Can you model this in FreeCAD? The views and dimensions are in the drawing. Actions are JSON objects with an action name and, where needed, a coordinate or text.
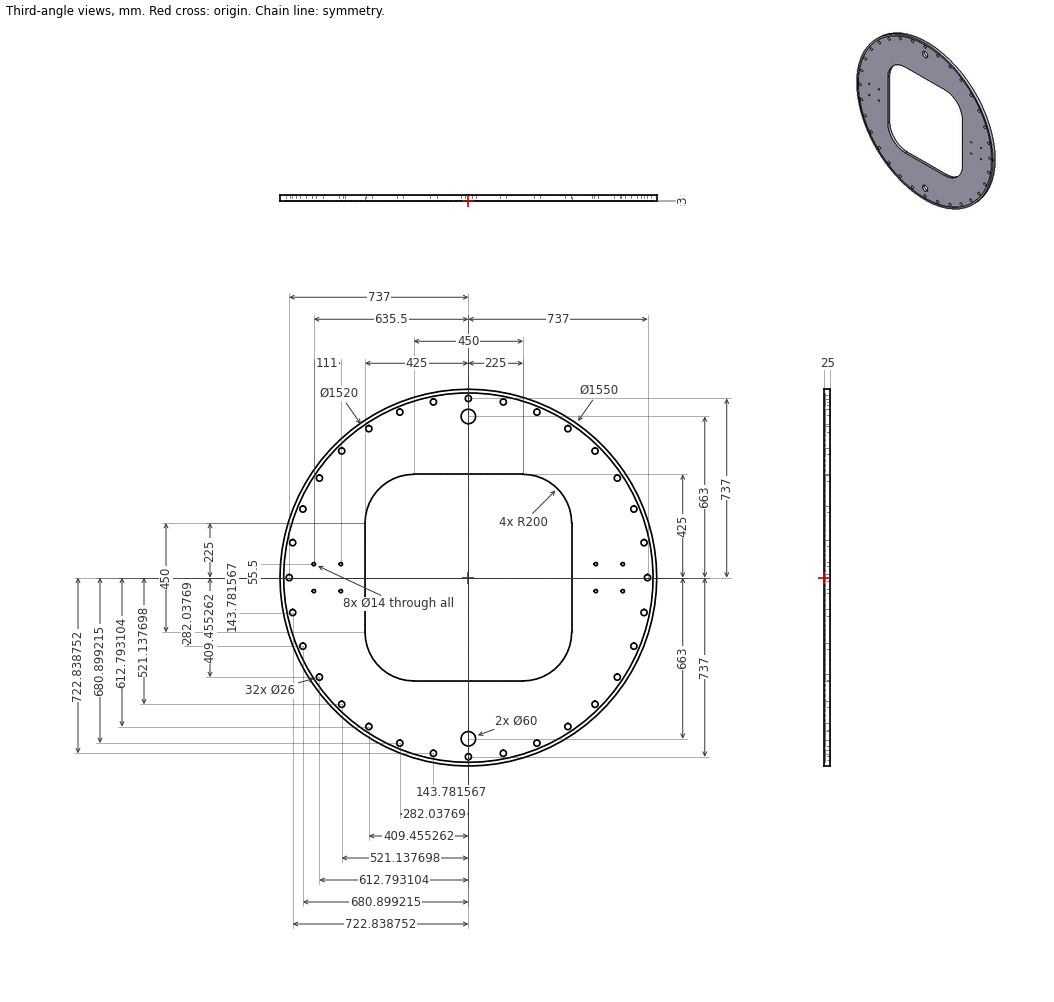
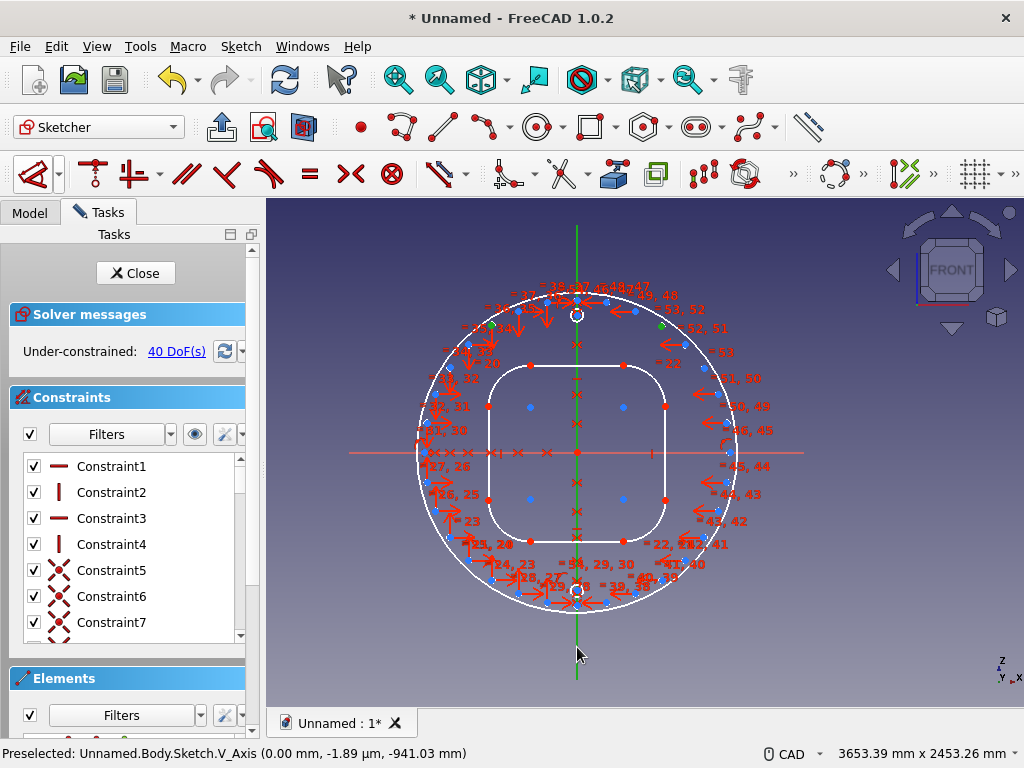
{"action": "left_click", "coordinate": [351, 174]}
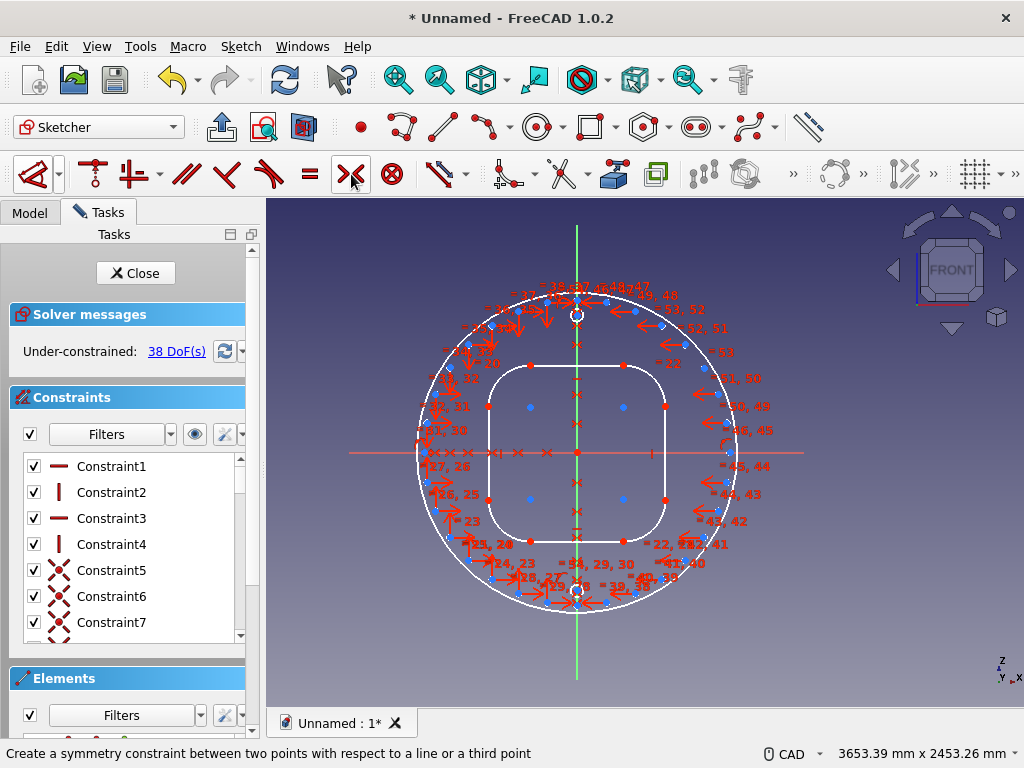
{"action": "left_click", "coordinate": [450, 368]}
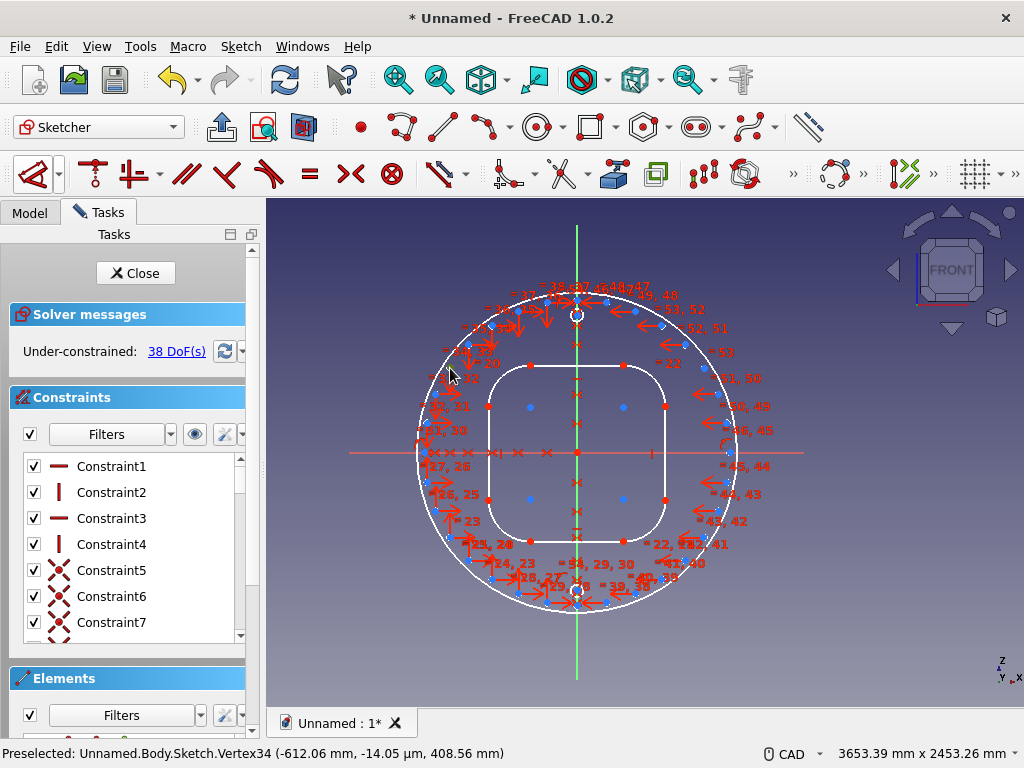
{"action": "left_click", "coordinate": [704, 368]}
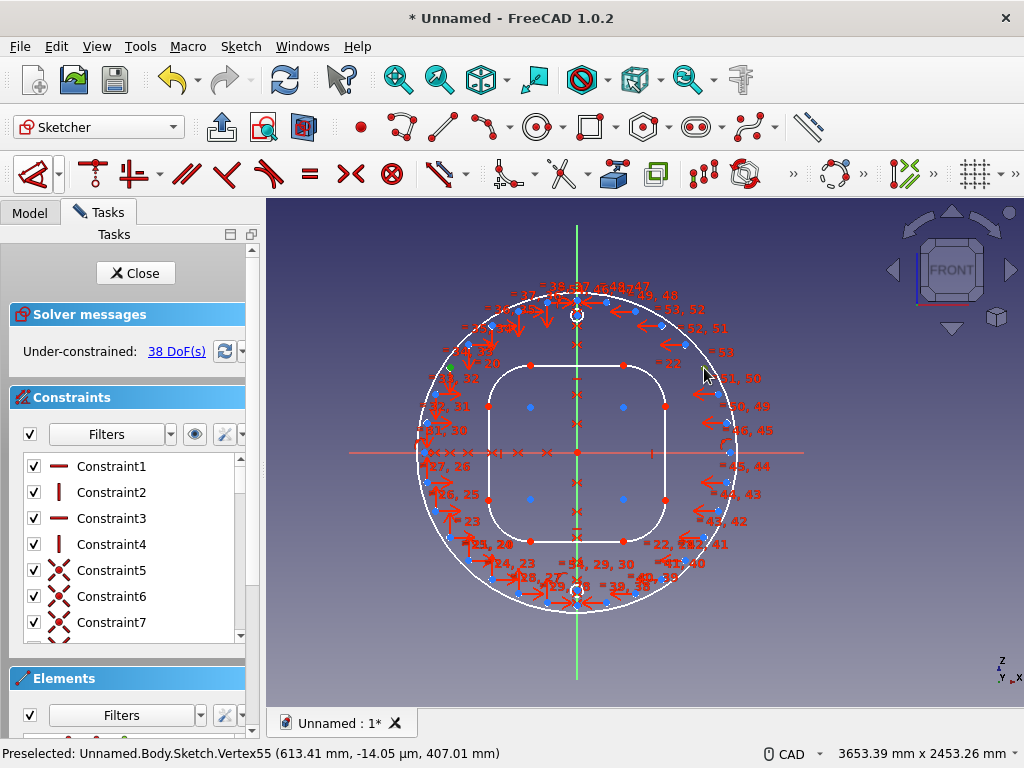
{"action": "left_click", "coordinate": [577, 647]}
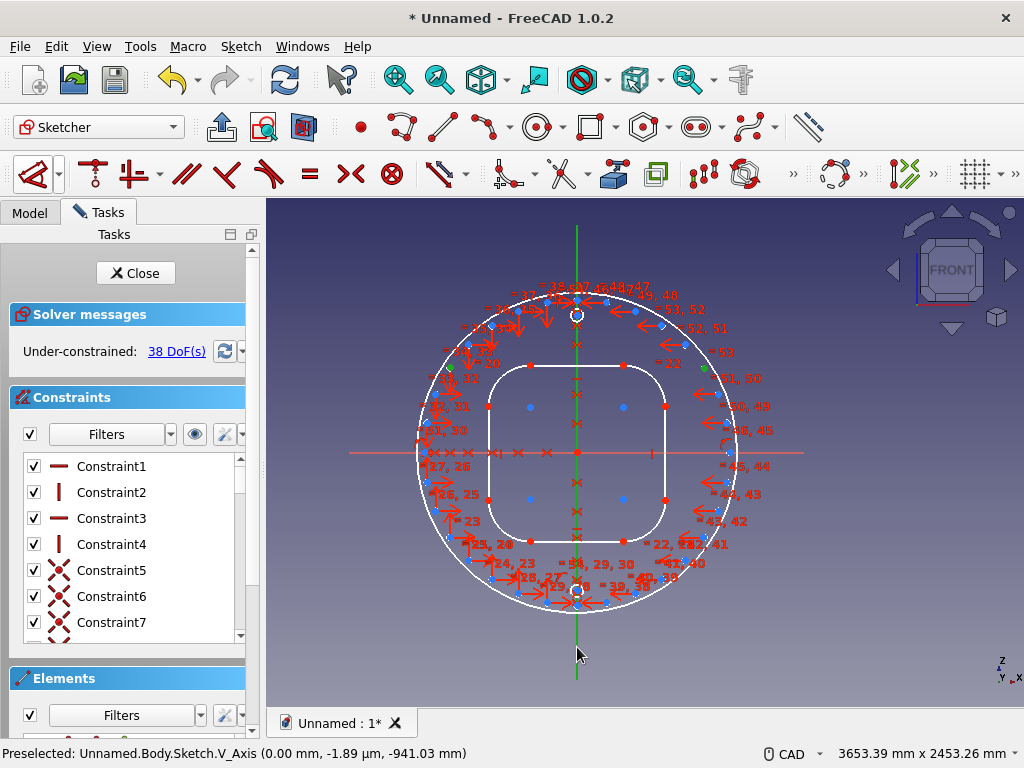
{"action": "left_click", "coordinate": [351, 174]}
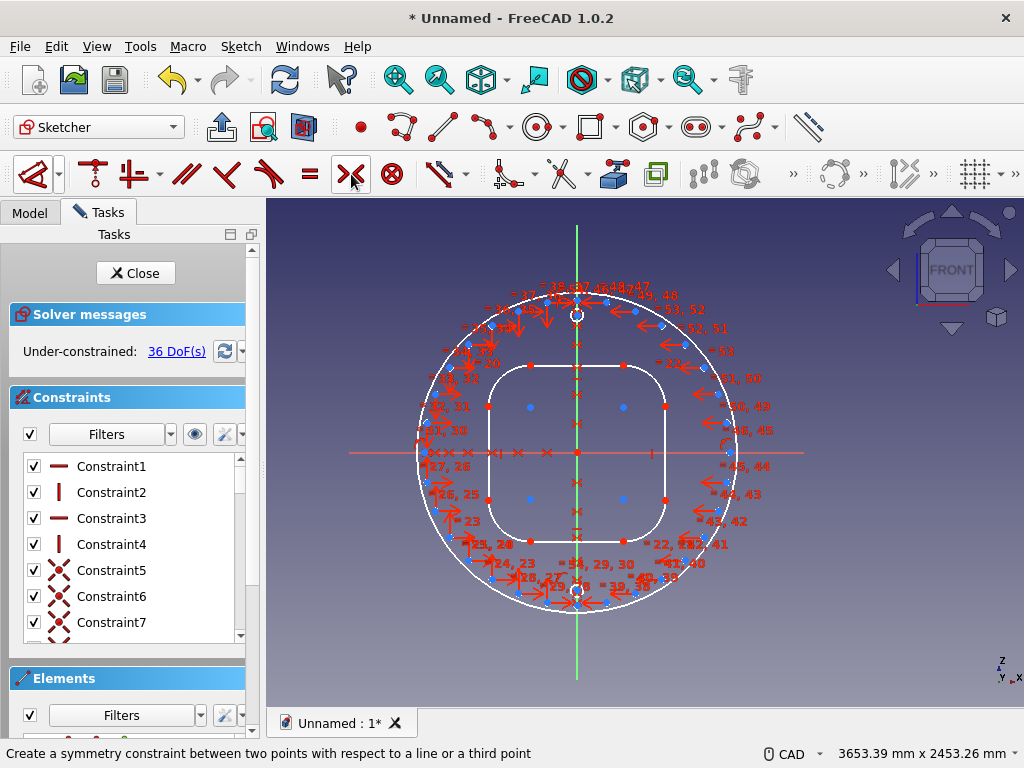
{"action": "left_click", "coordinate": [530, 366]}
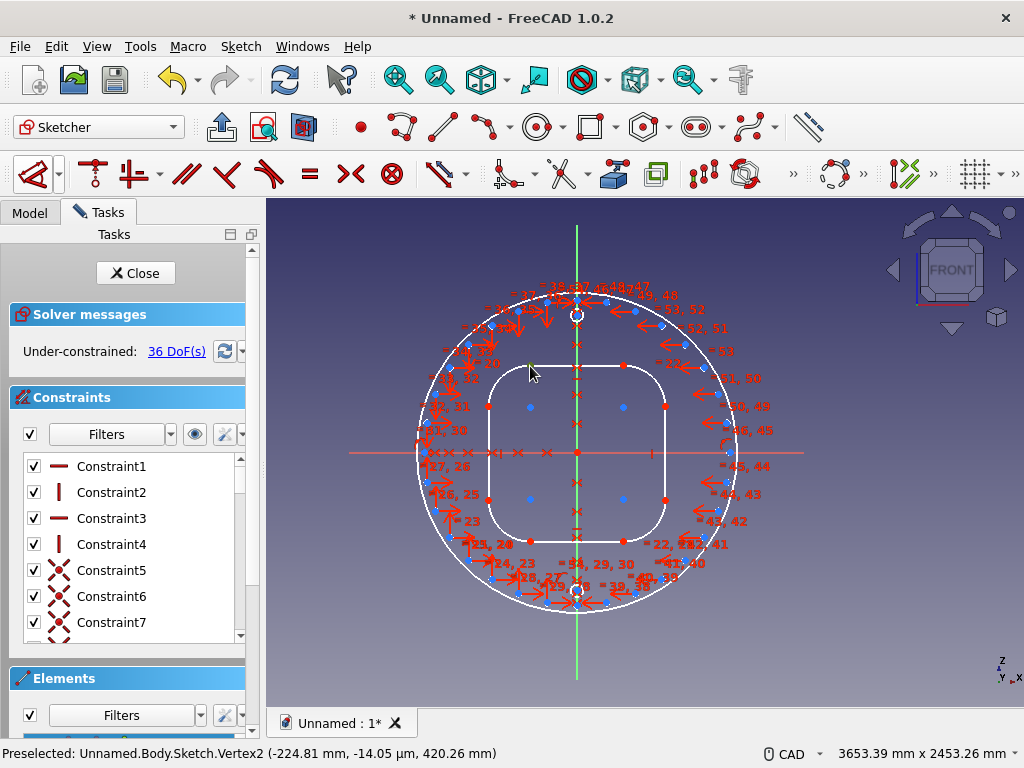
{"action": "left_click", "coordinate": [530, 542]}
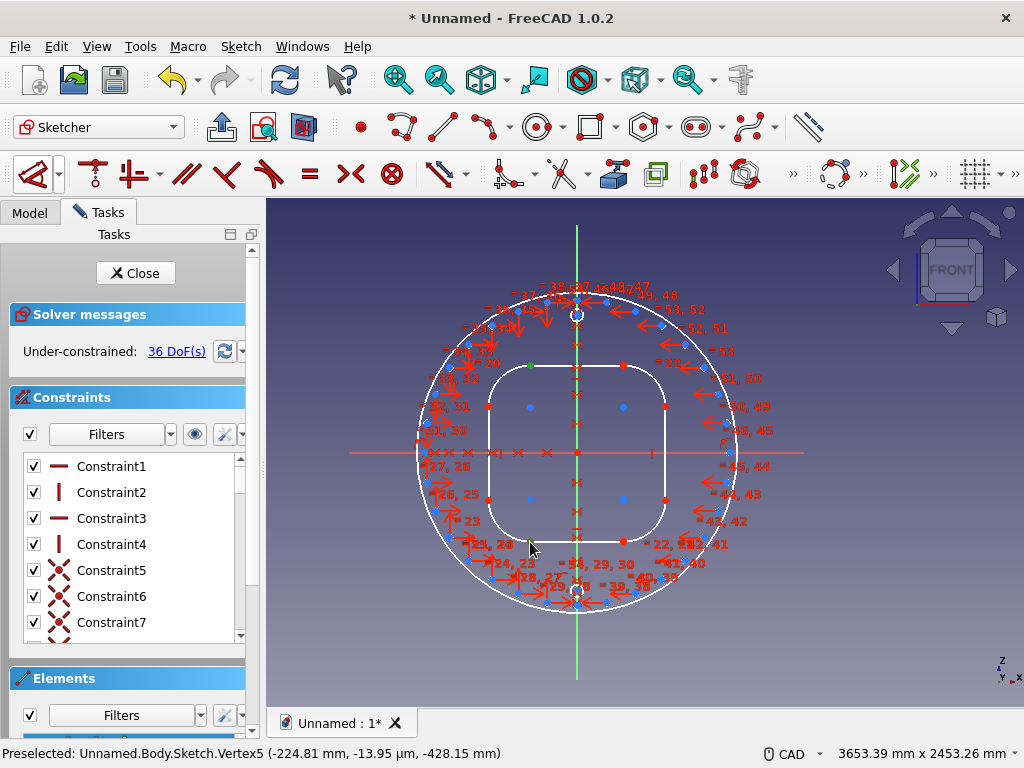
{"action": "left_click", "coordinate": [375, 453]}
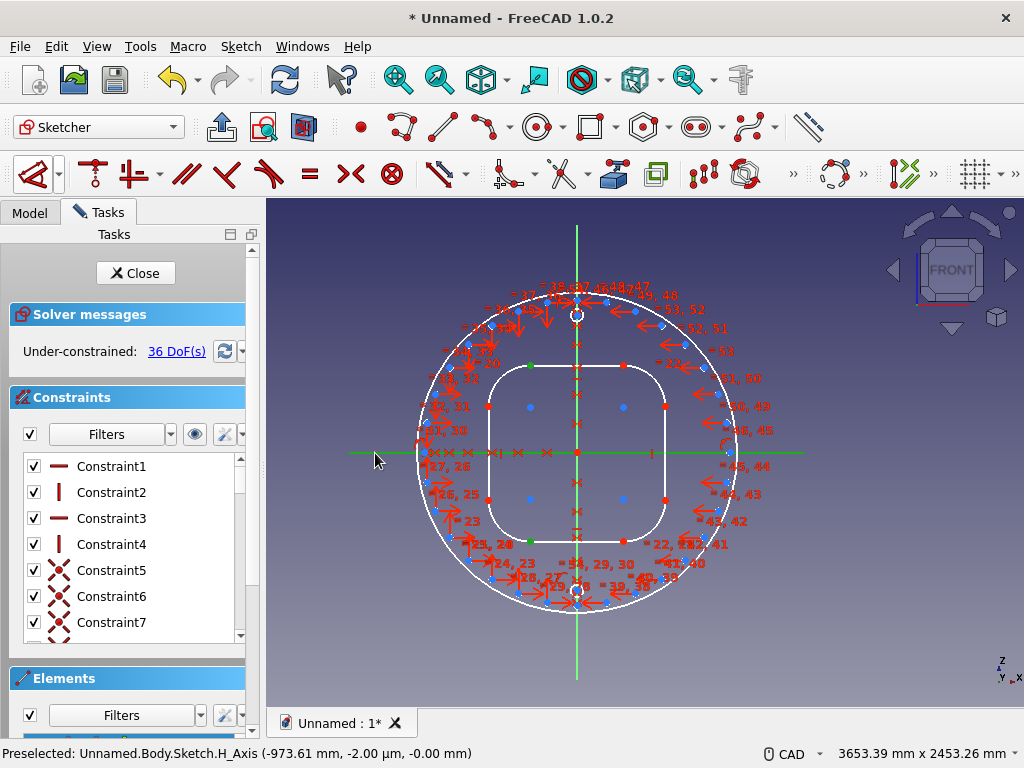
{"action": "left_click", "coordinate": [351, 174]}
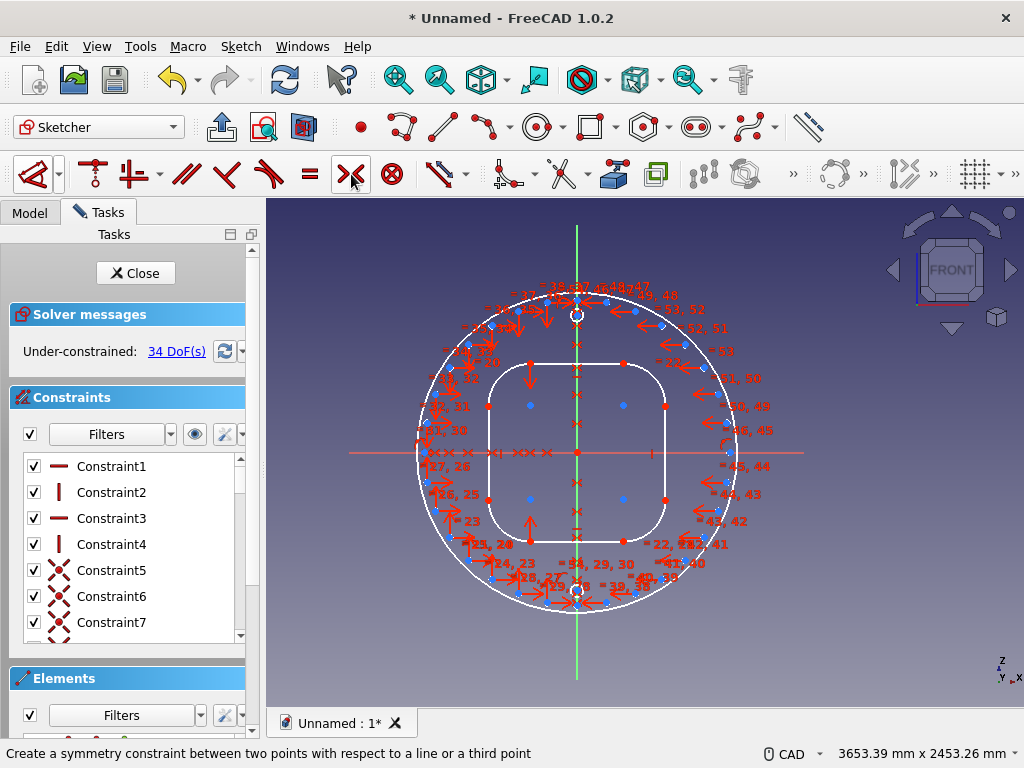
{"action": "left_click", "coordinate": [489, 501]}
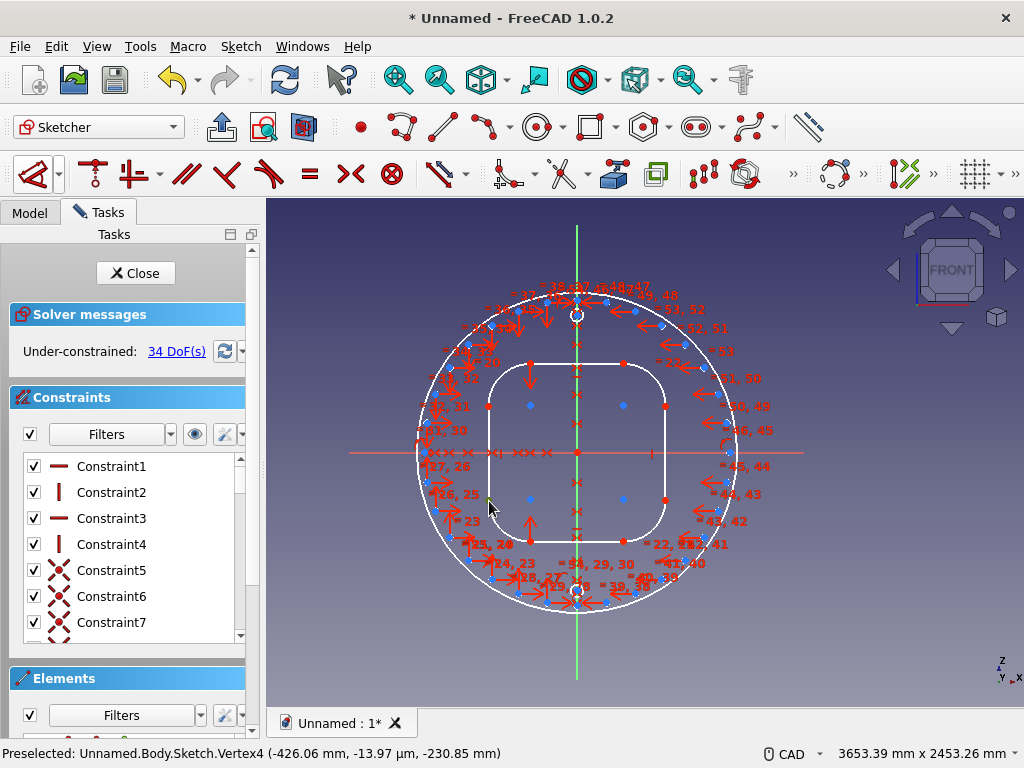
{"action": "left_click", "coordinate": [665, 501]}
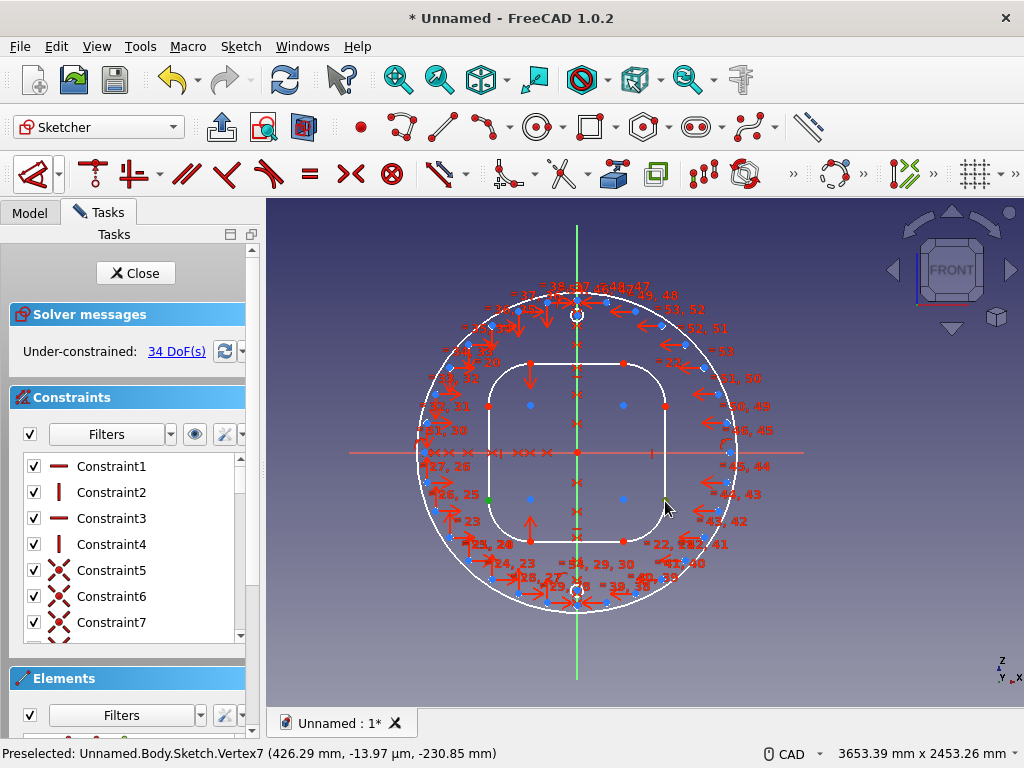
{"action": "left_click", "coordinate": [577, 647]}